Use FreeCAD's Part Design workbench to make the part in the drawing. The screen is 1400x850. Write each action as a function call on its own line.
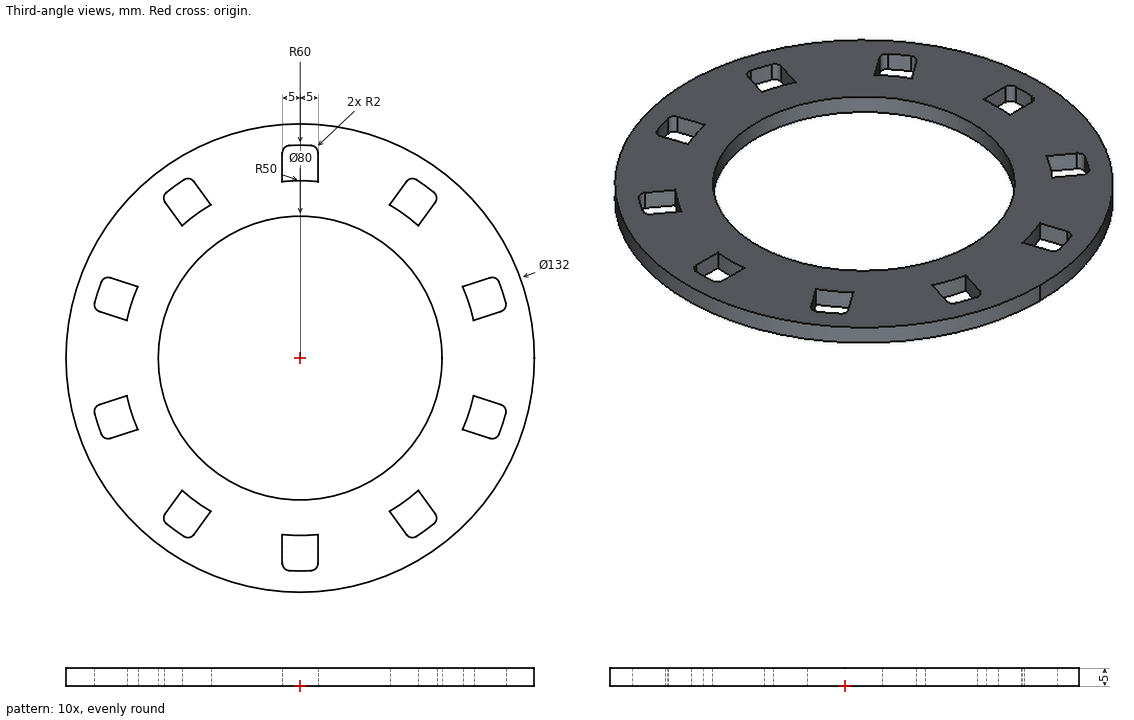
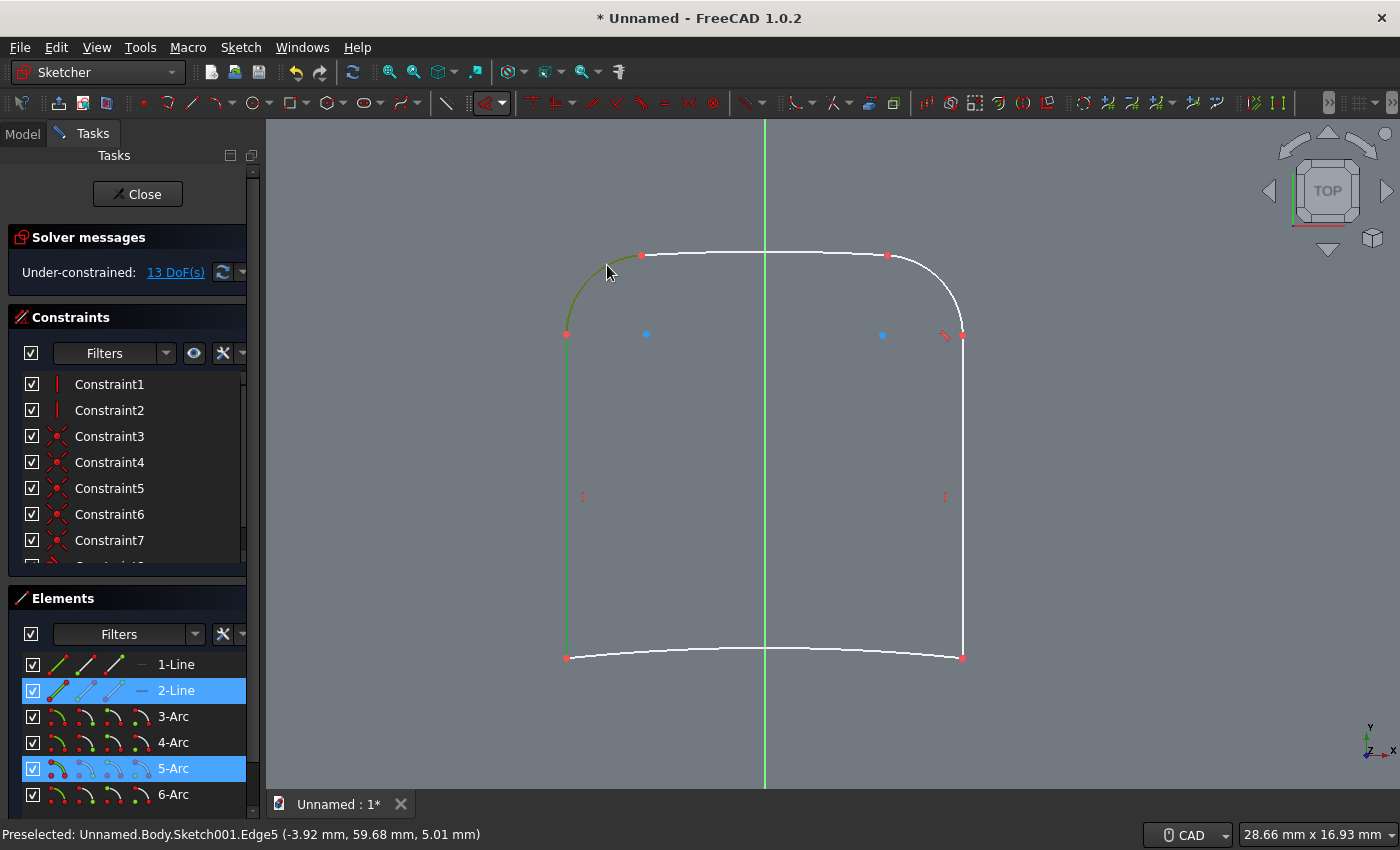
key(t)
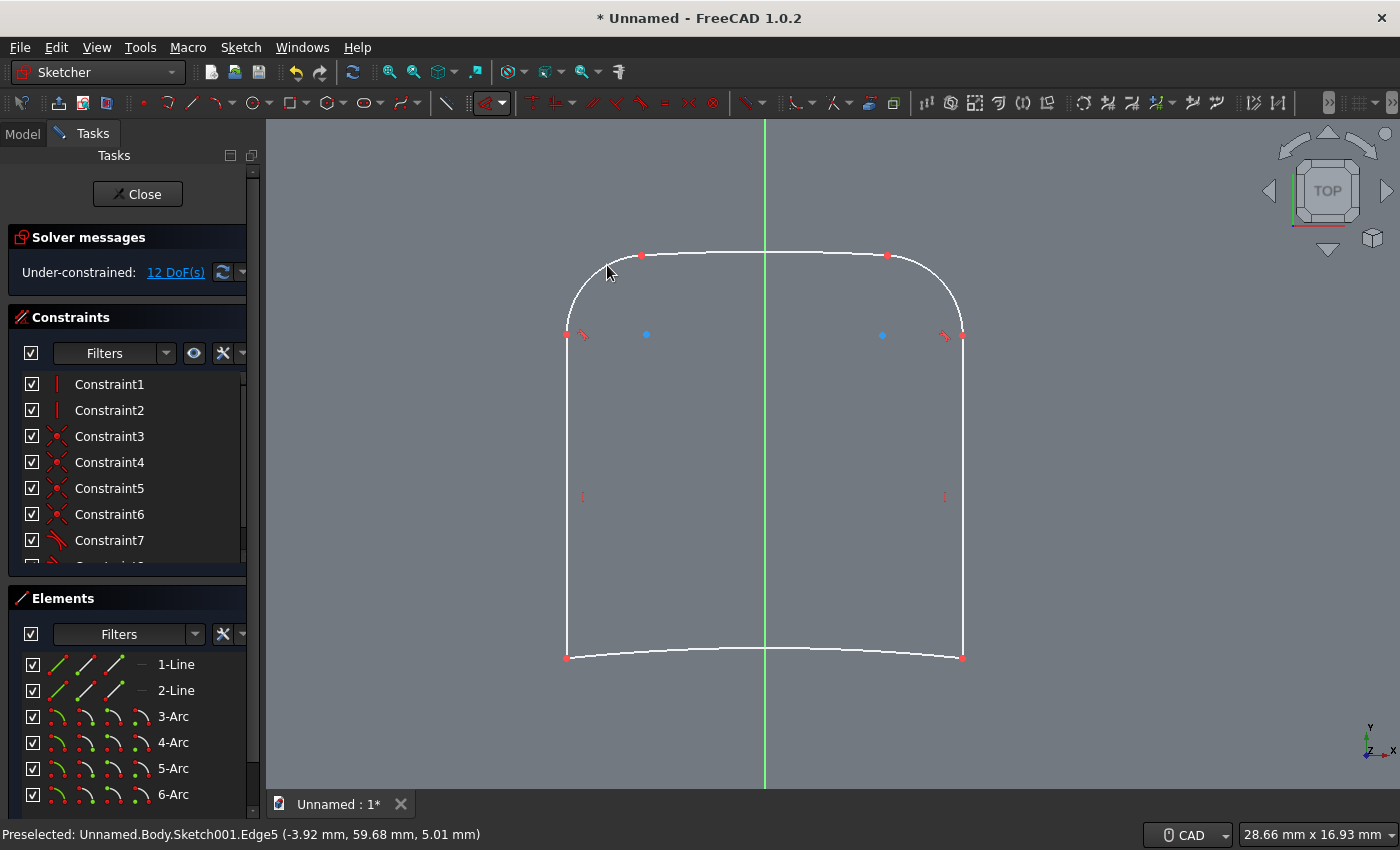
click(955, 301)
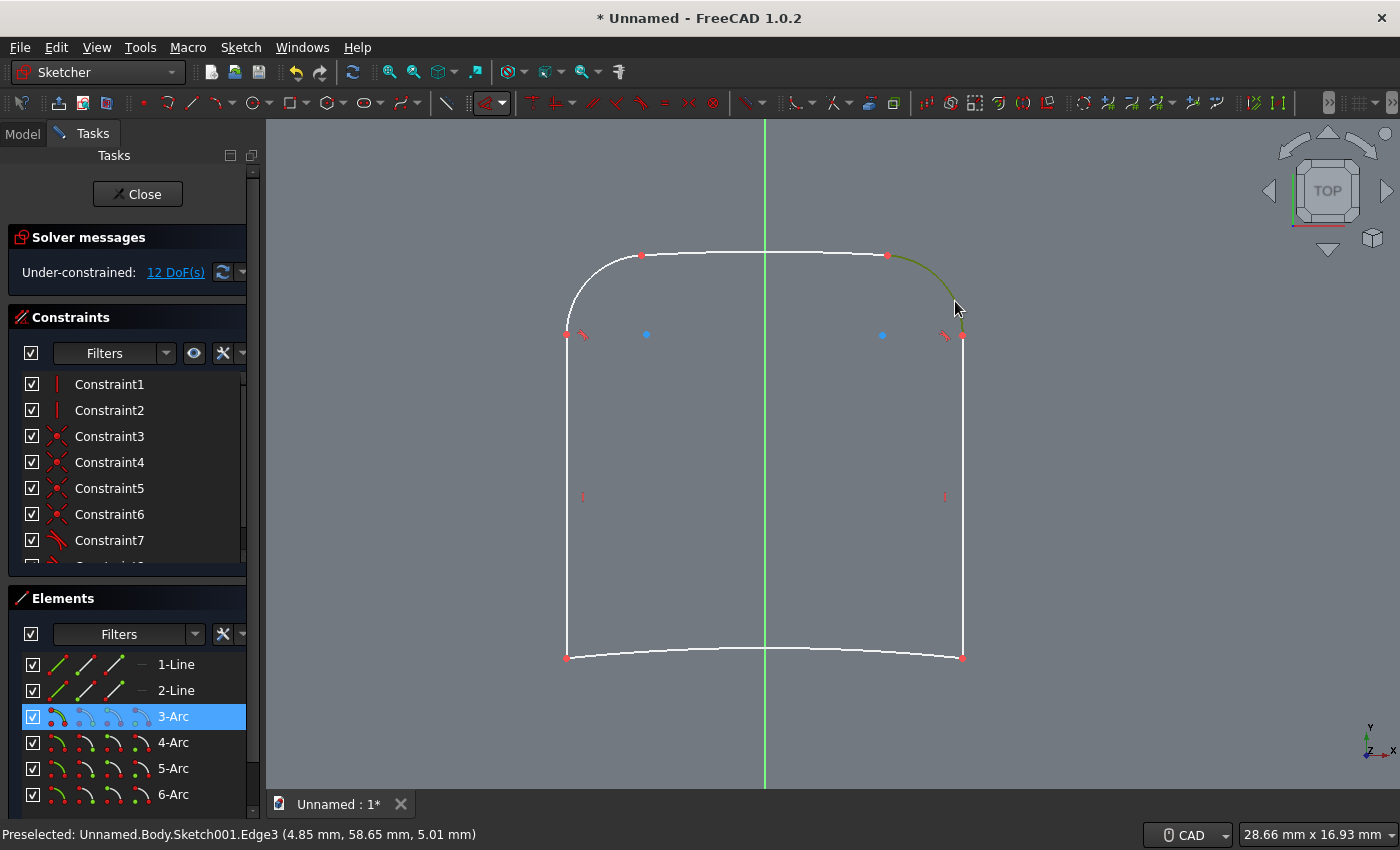
click(814, 252)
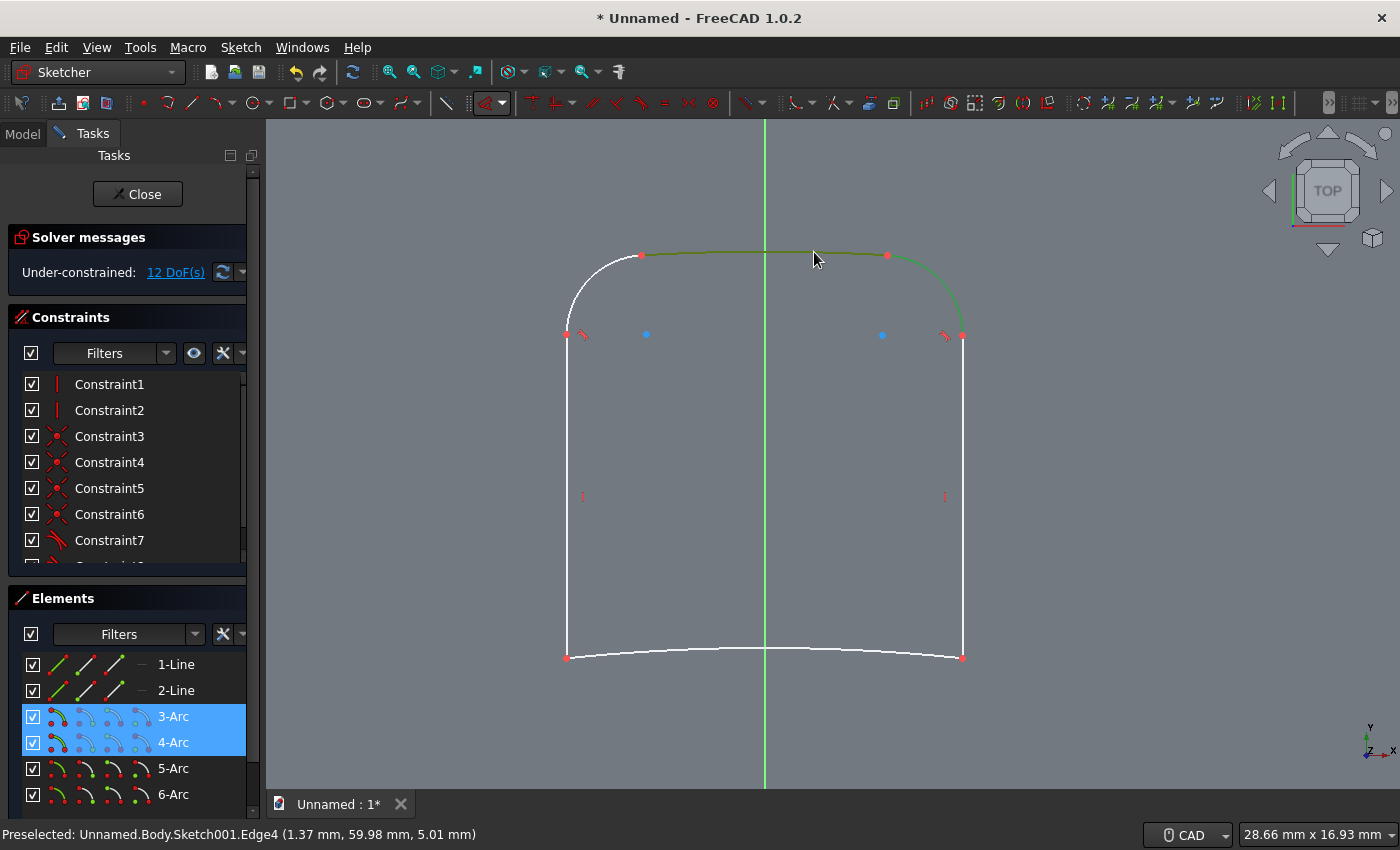
key(t)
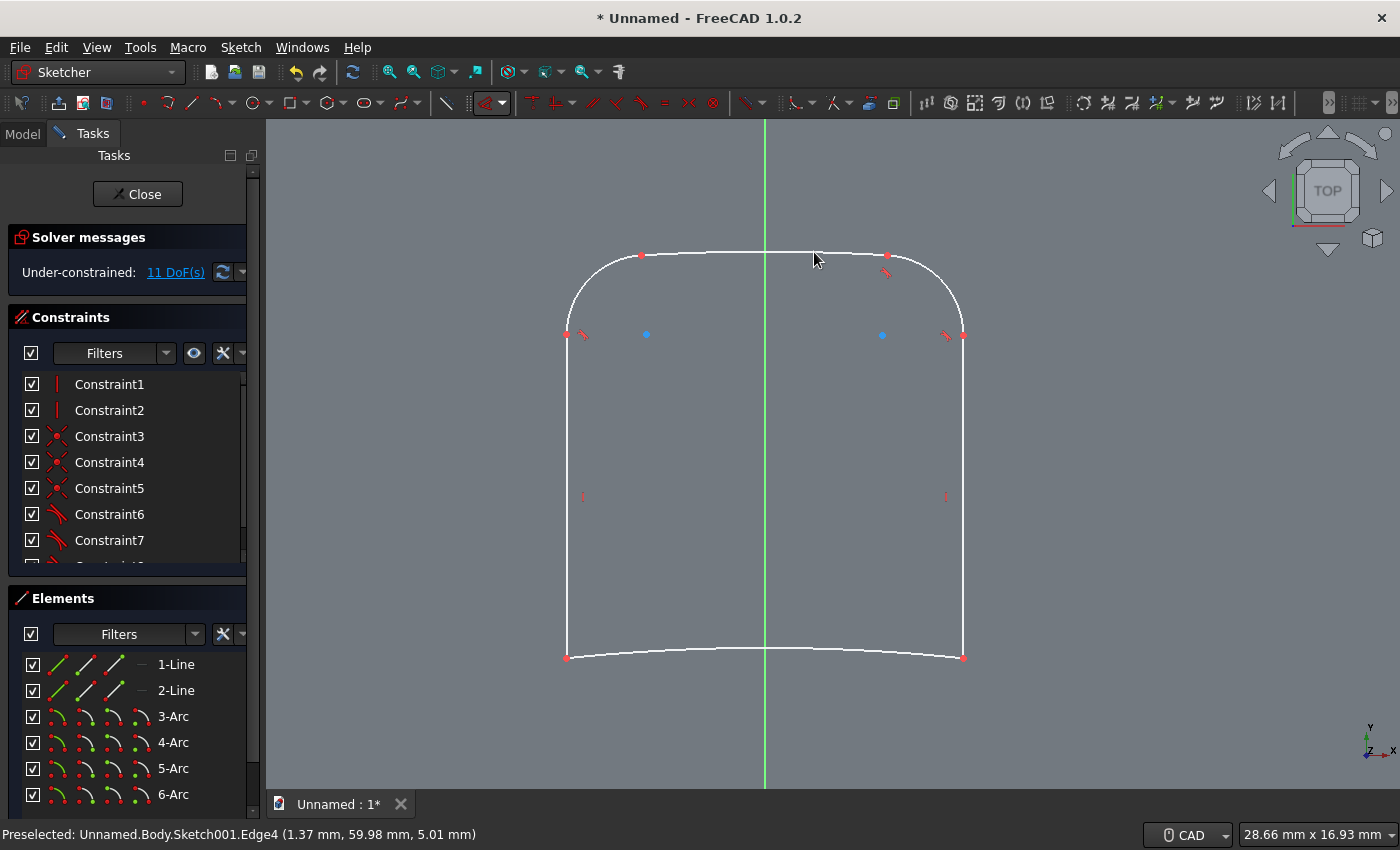
click(814, 252)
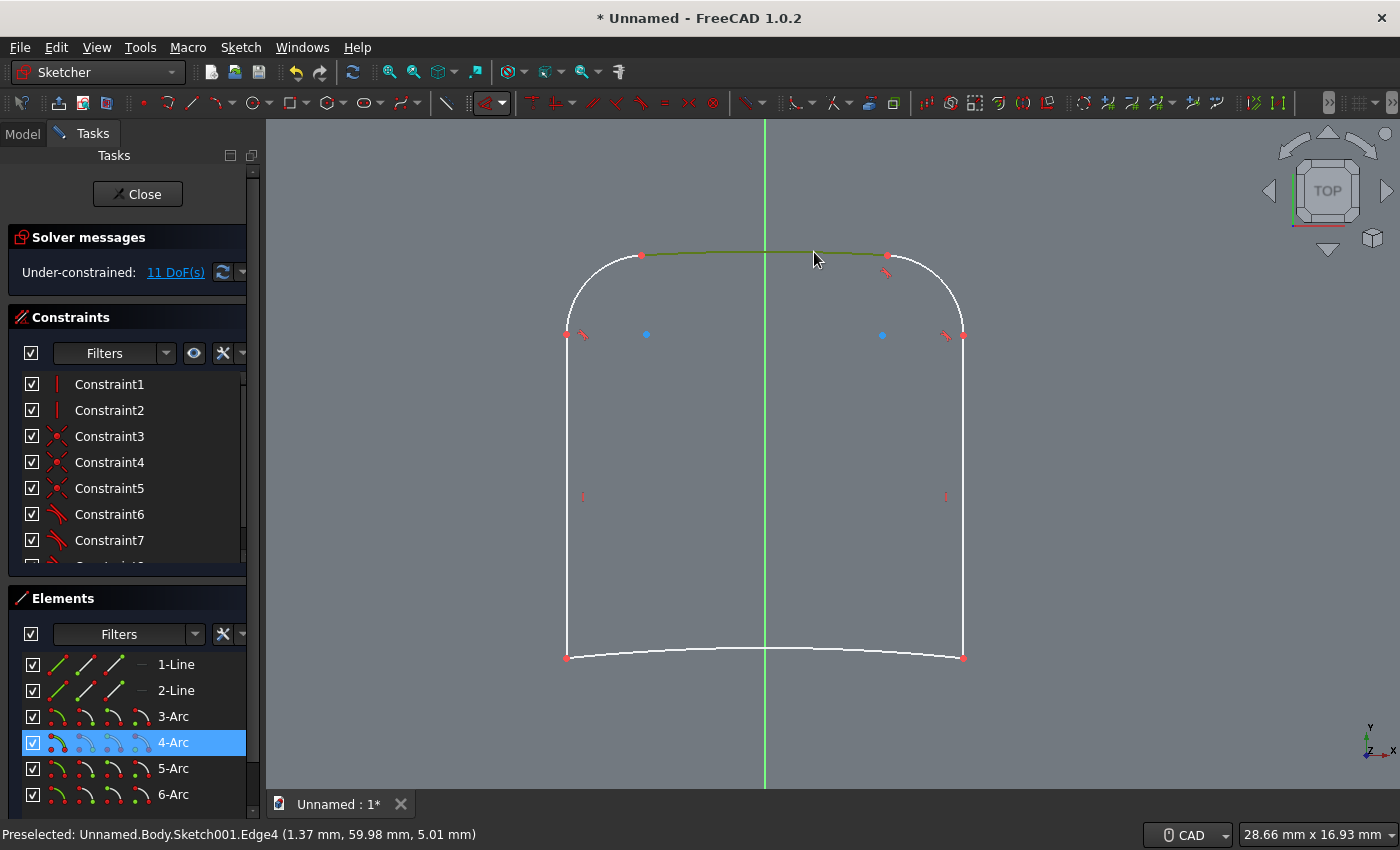
click(607, 265)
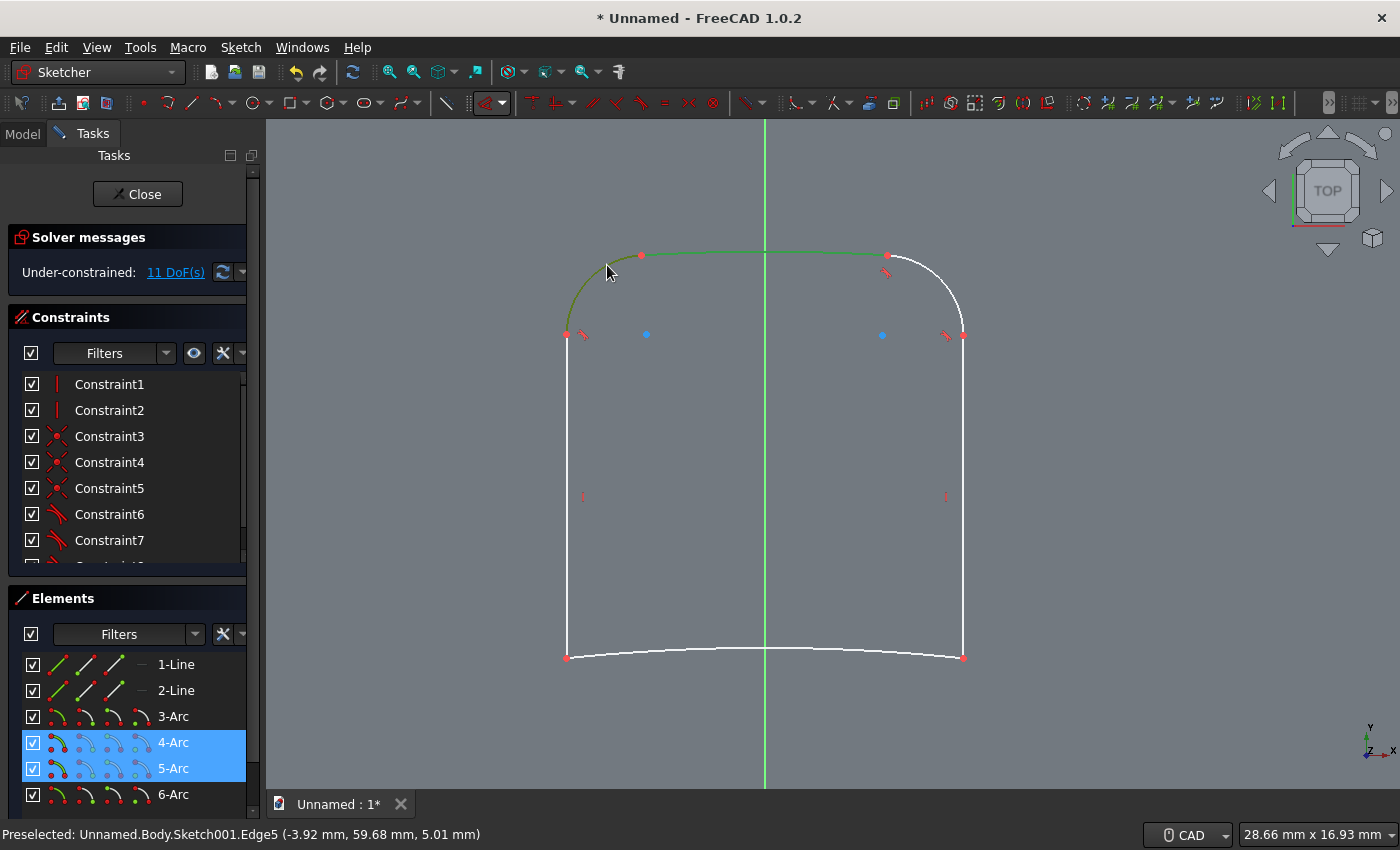
click(642, 104)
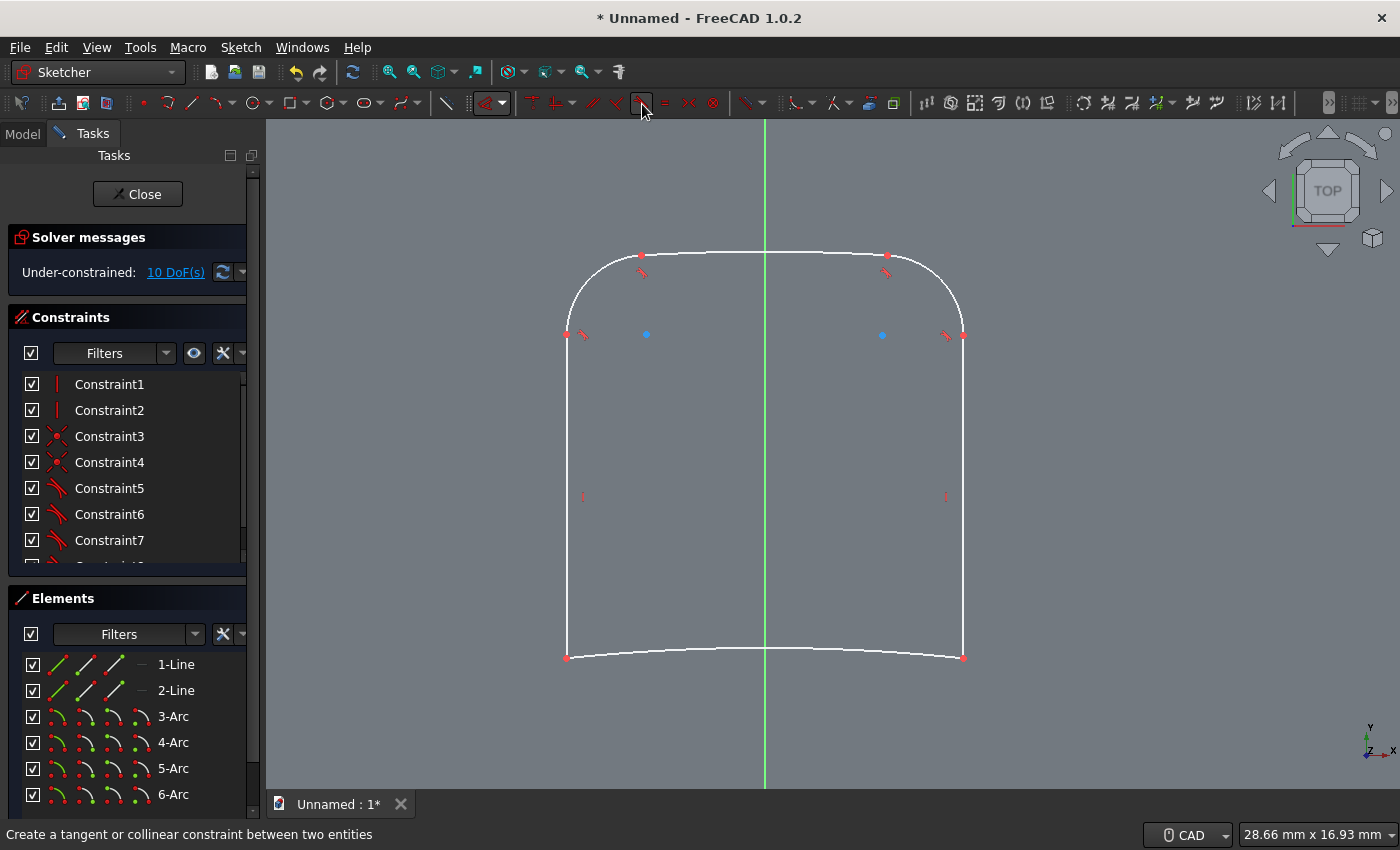
click(814, 252)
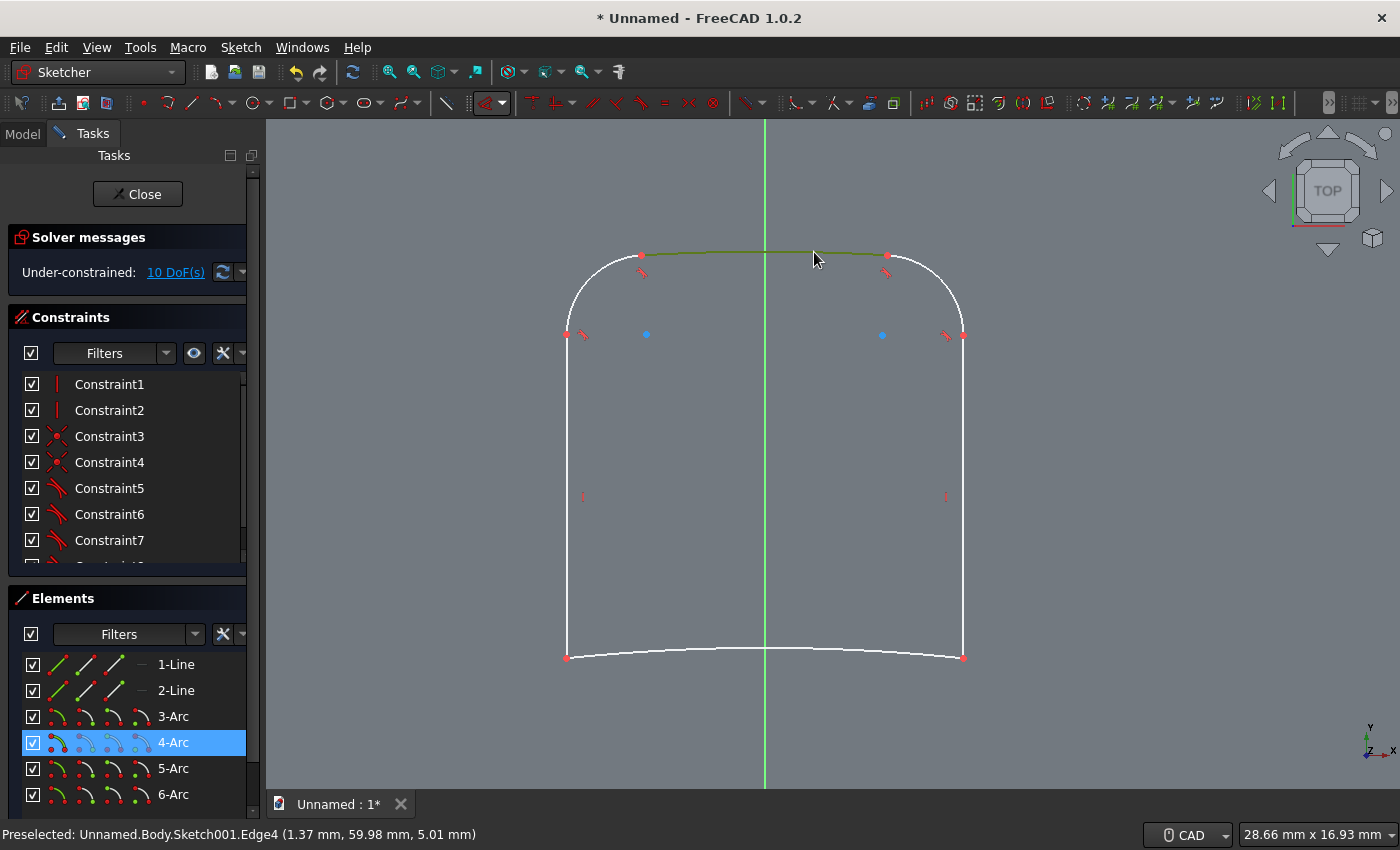
click(845, 650)